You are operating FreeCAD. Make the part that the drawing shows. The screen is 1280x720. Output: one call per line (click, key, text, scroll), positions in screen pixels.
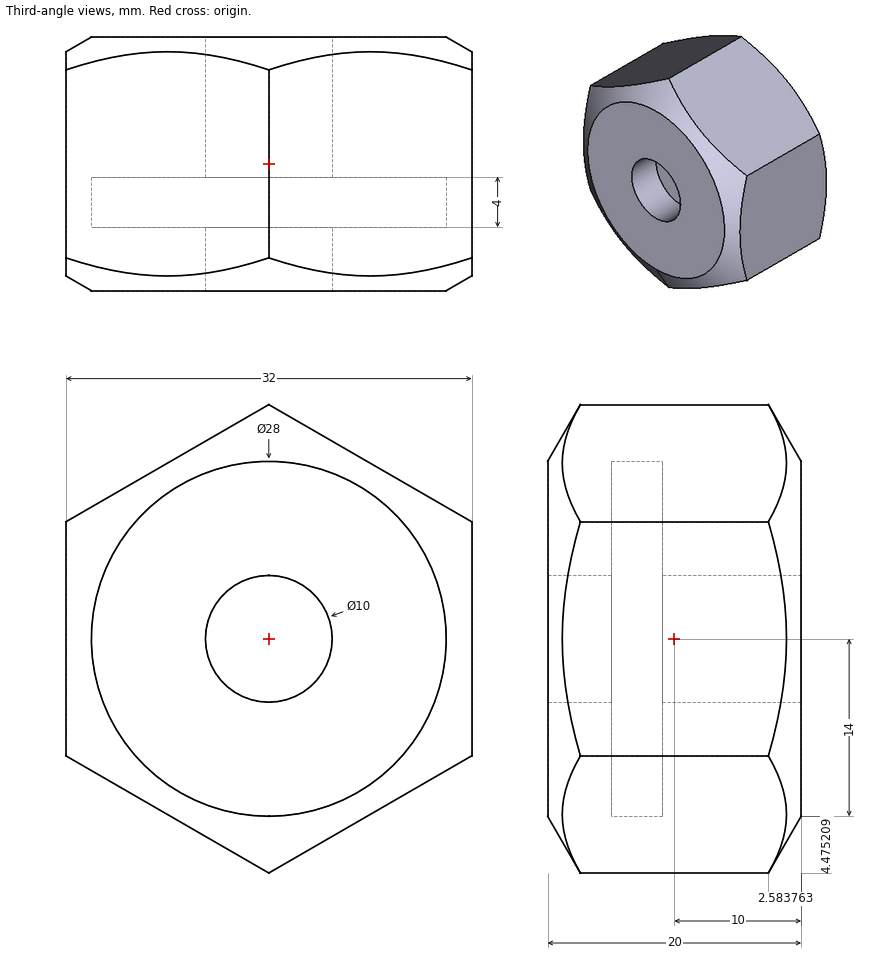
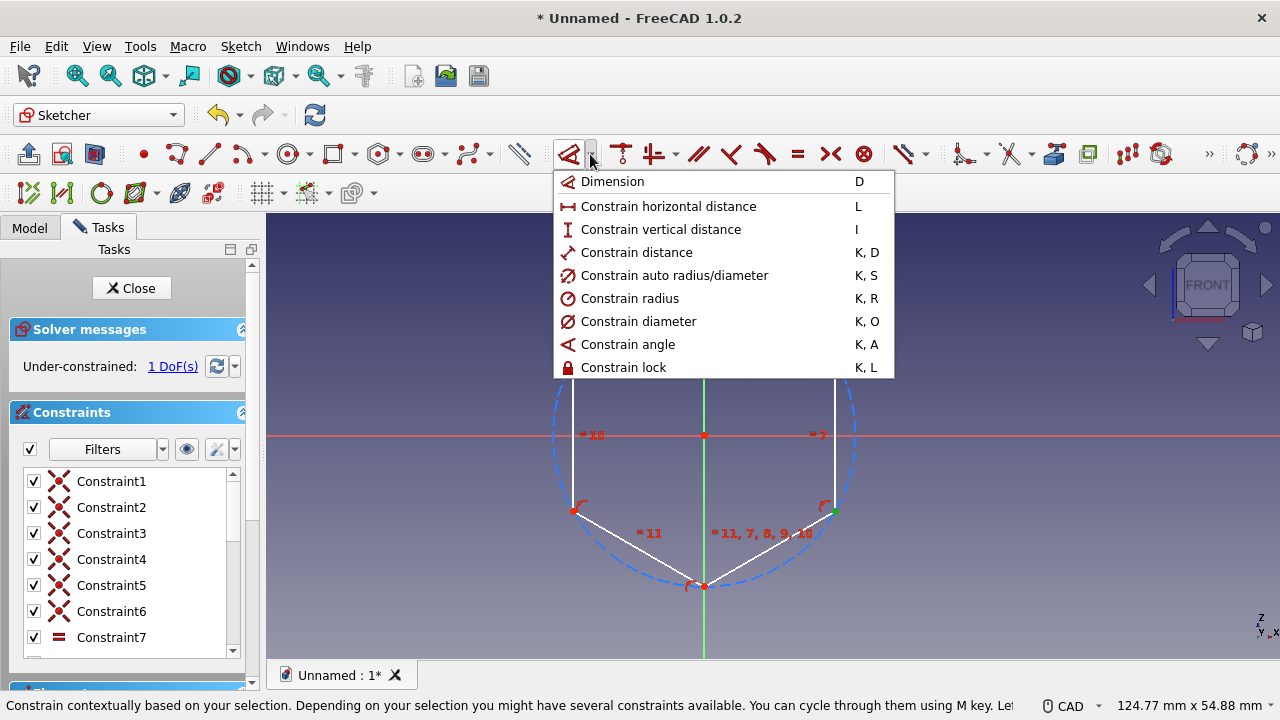
click(724, 206)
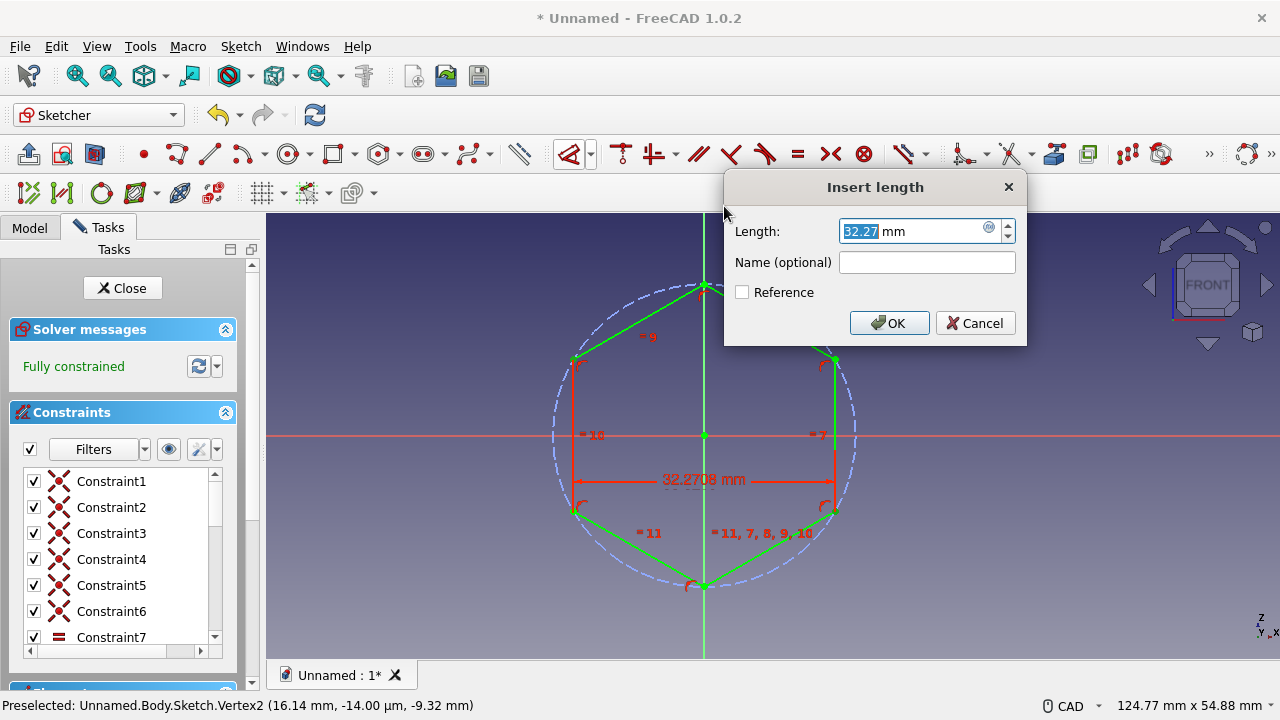
text(32)
key(Return)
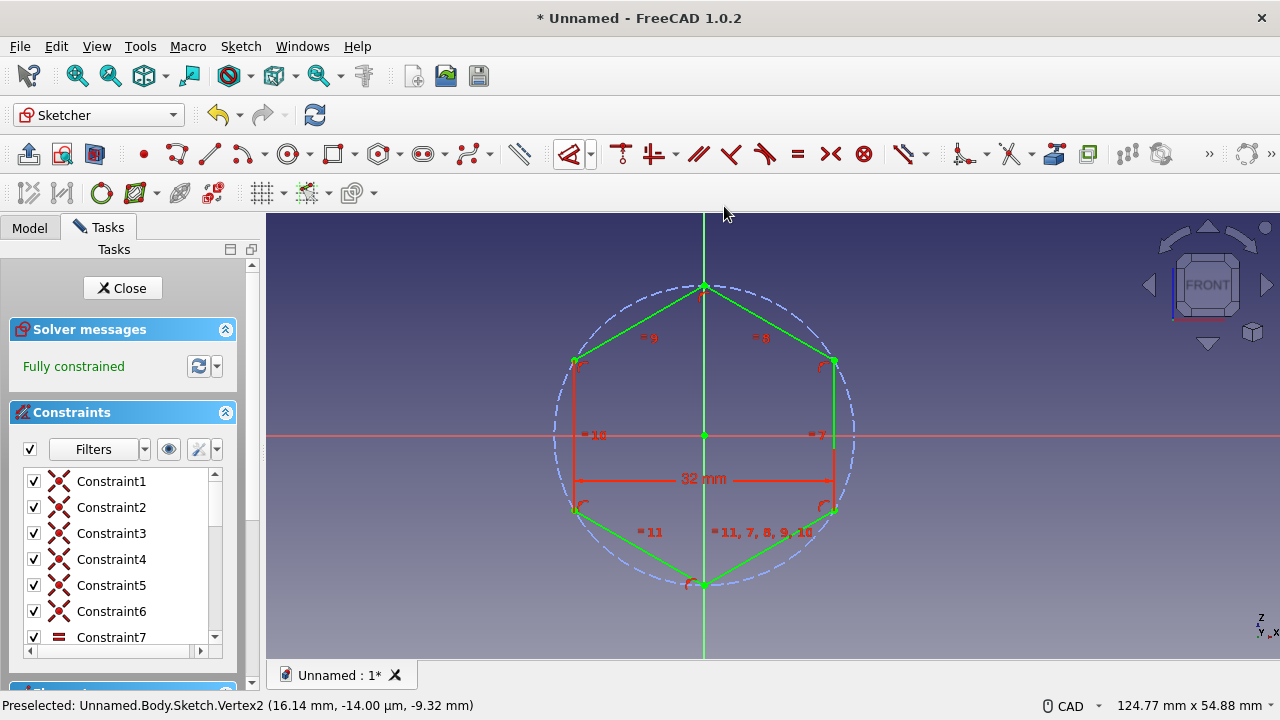
click(123, 288)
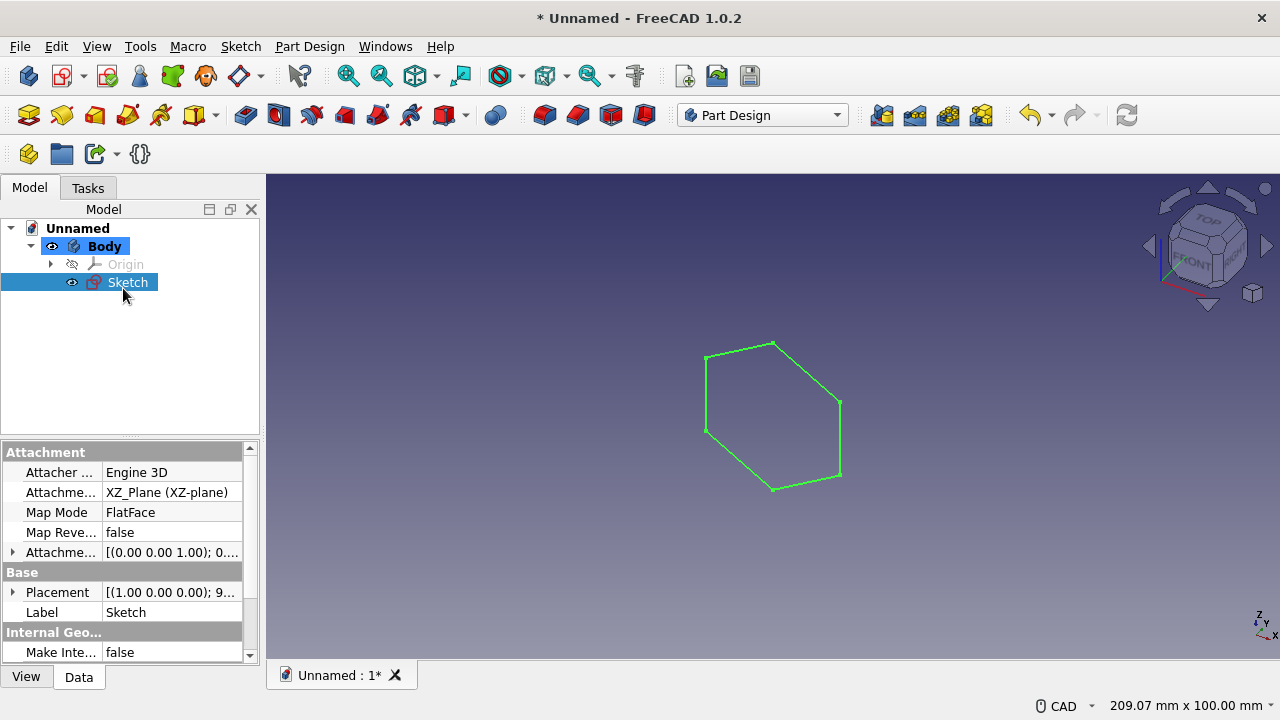
click(29, 116)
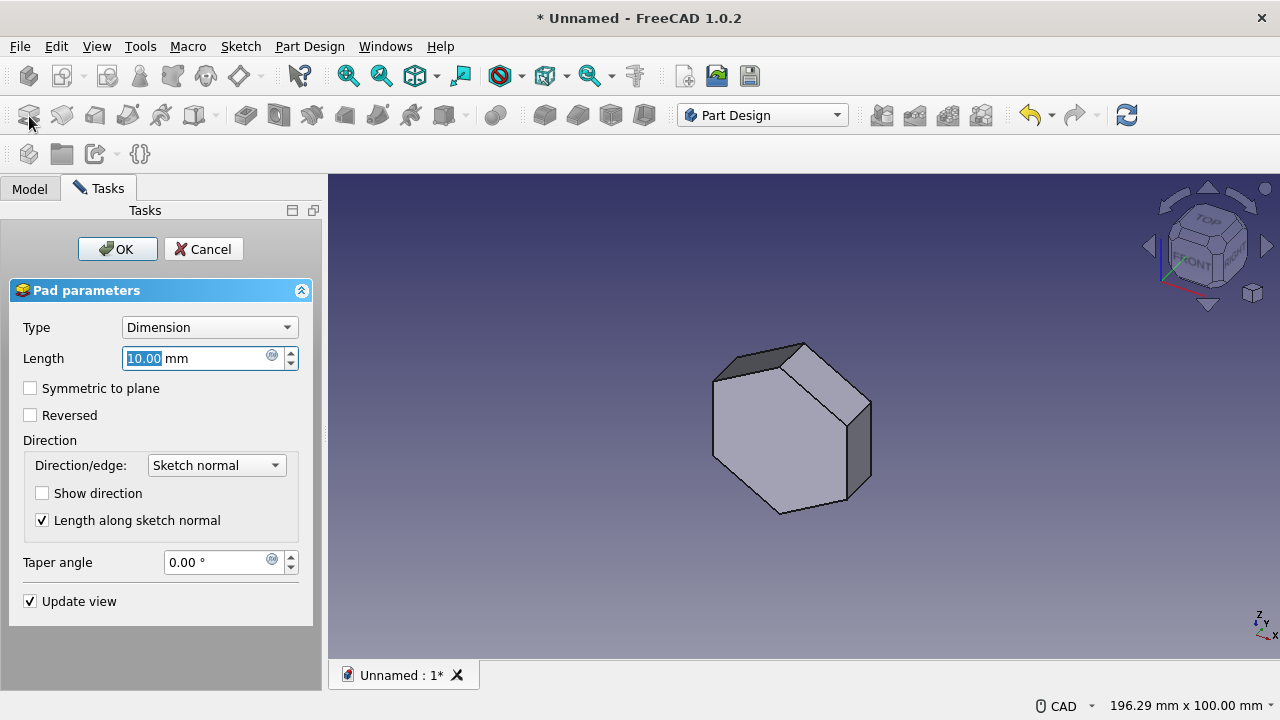
text(20)
key(Tab)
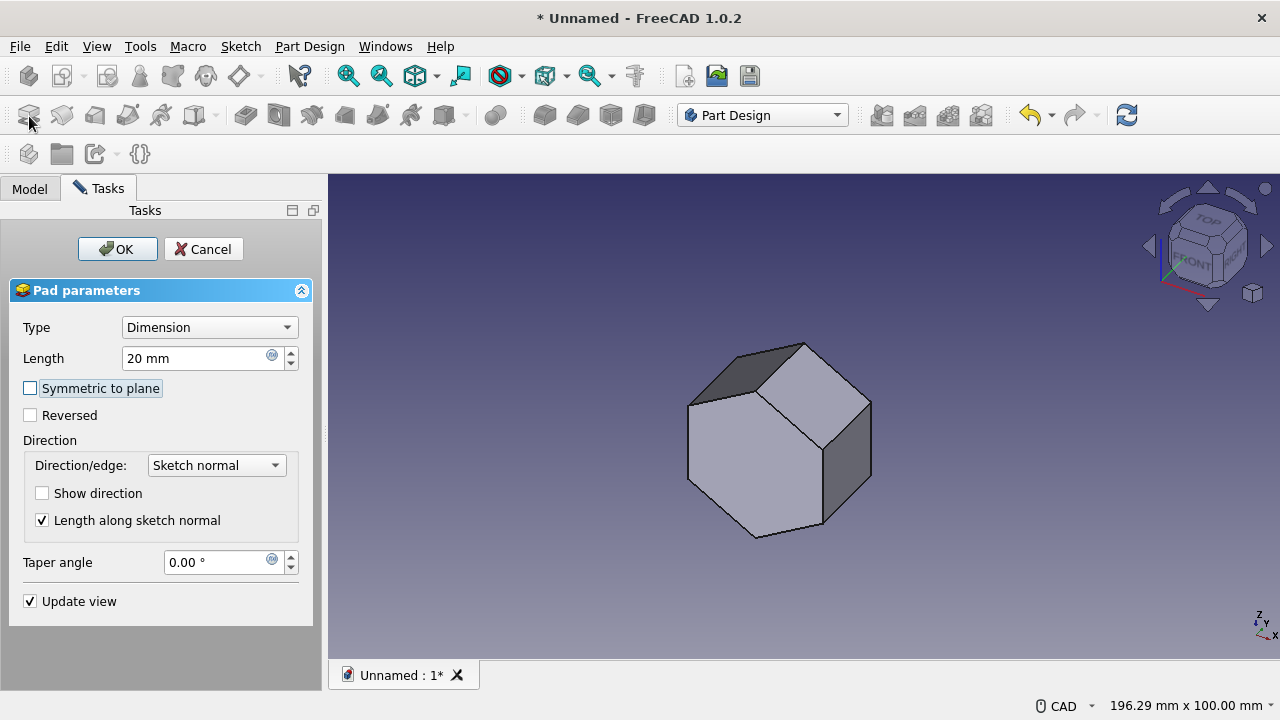
click(31, 388)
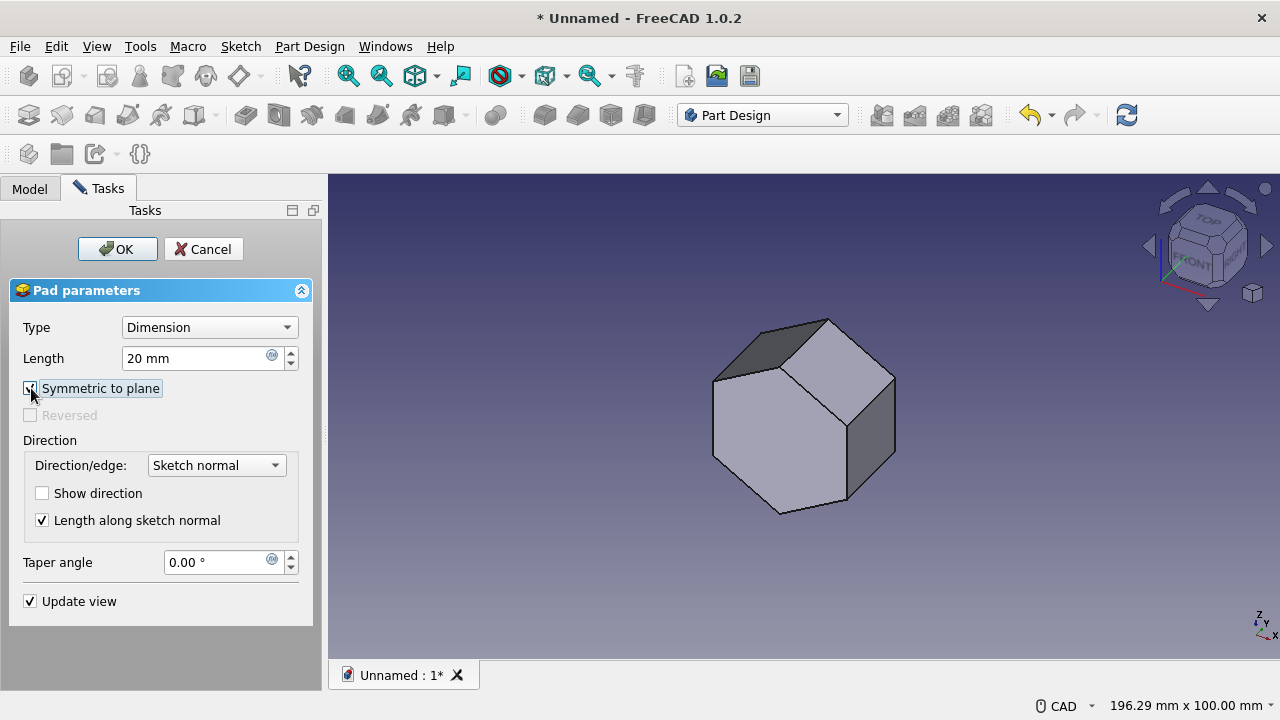
click(118, 249)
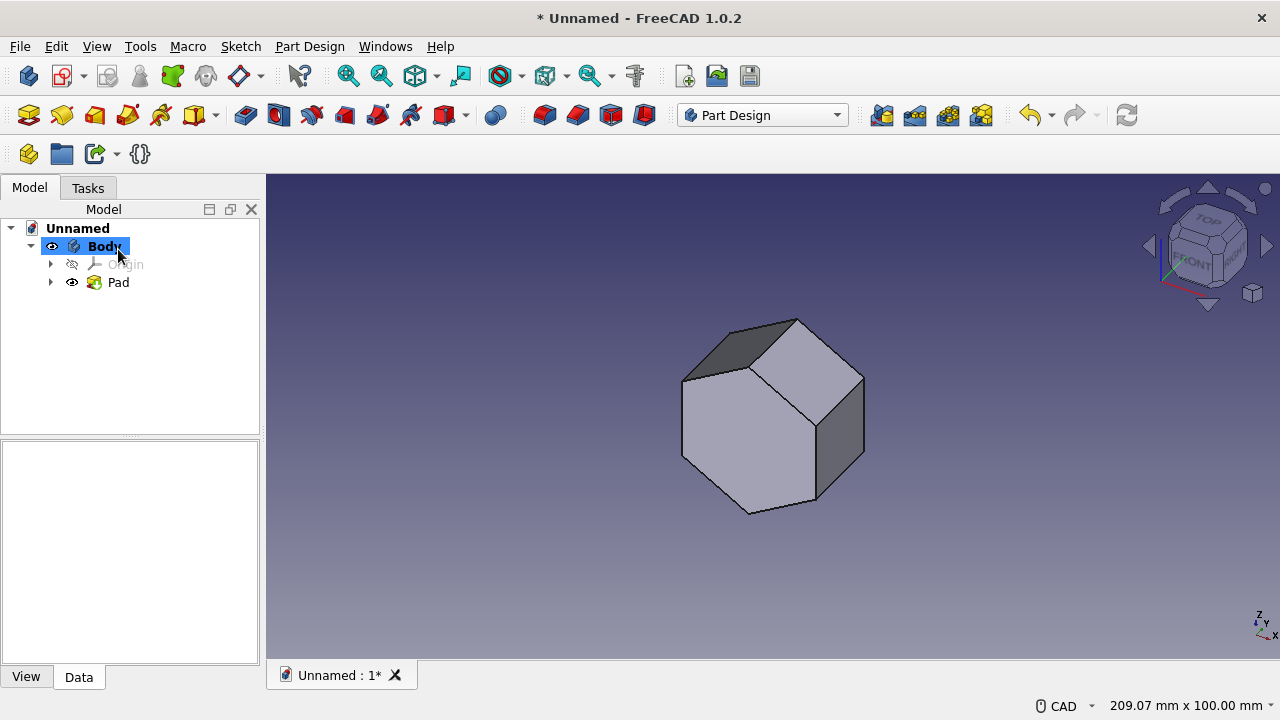
key(4)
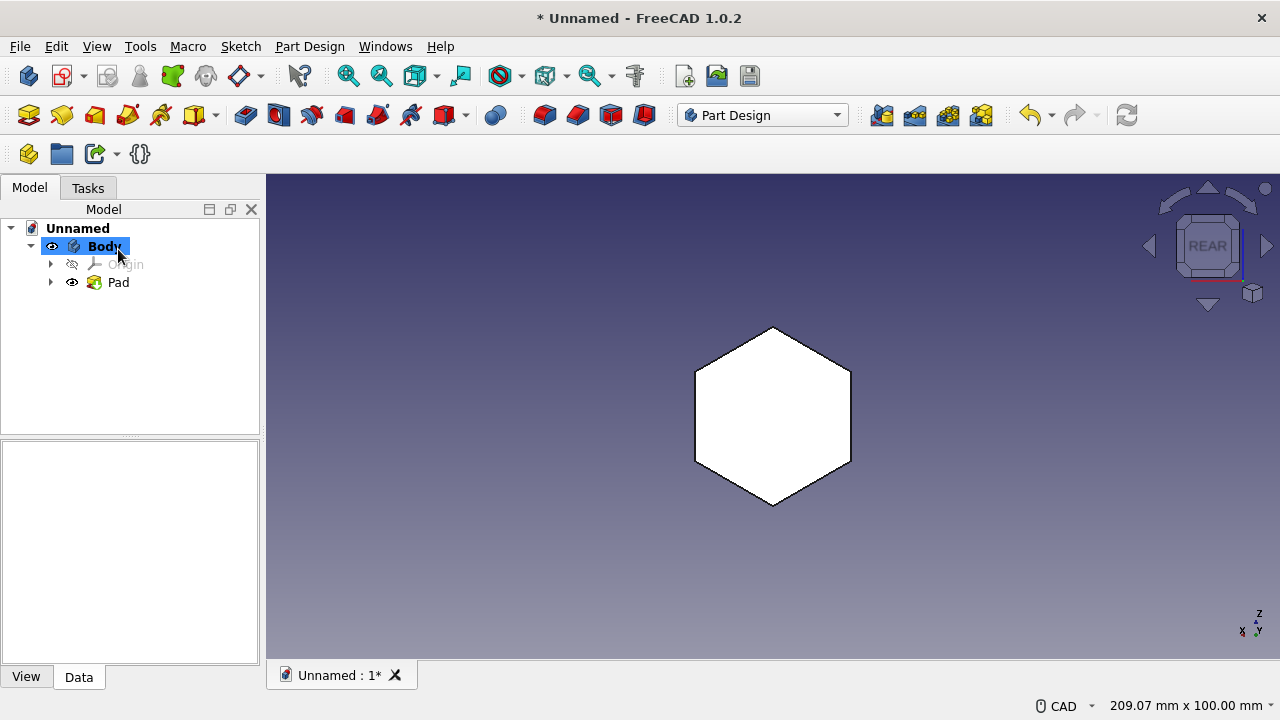
click(349, 76)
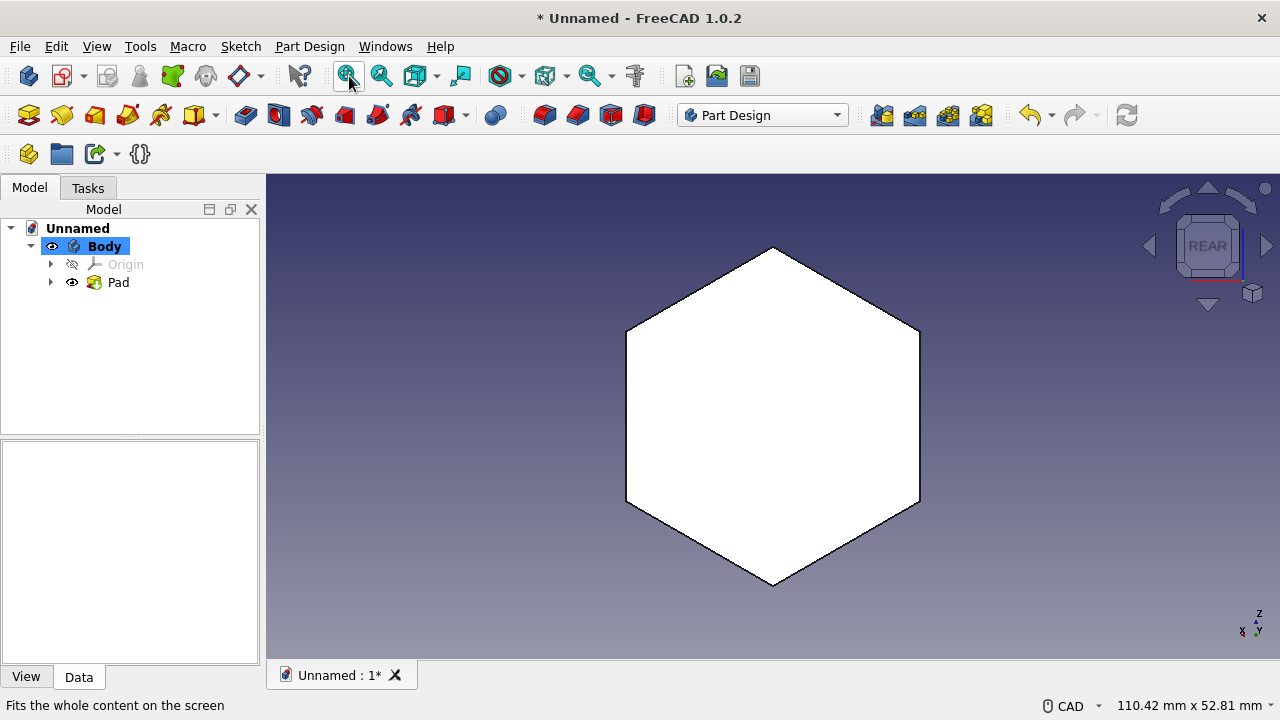
click(773, 416)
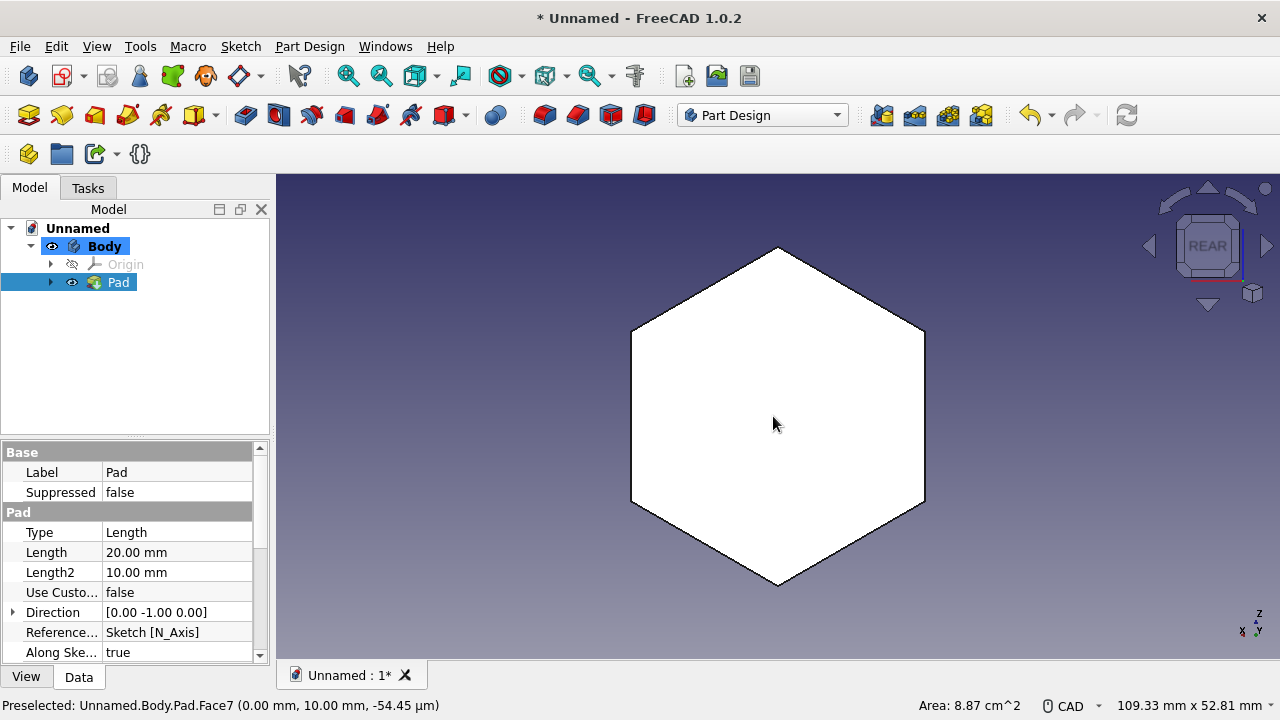
click(62, 76)